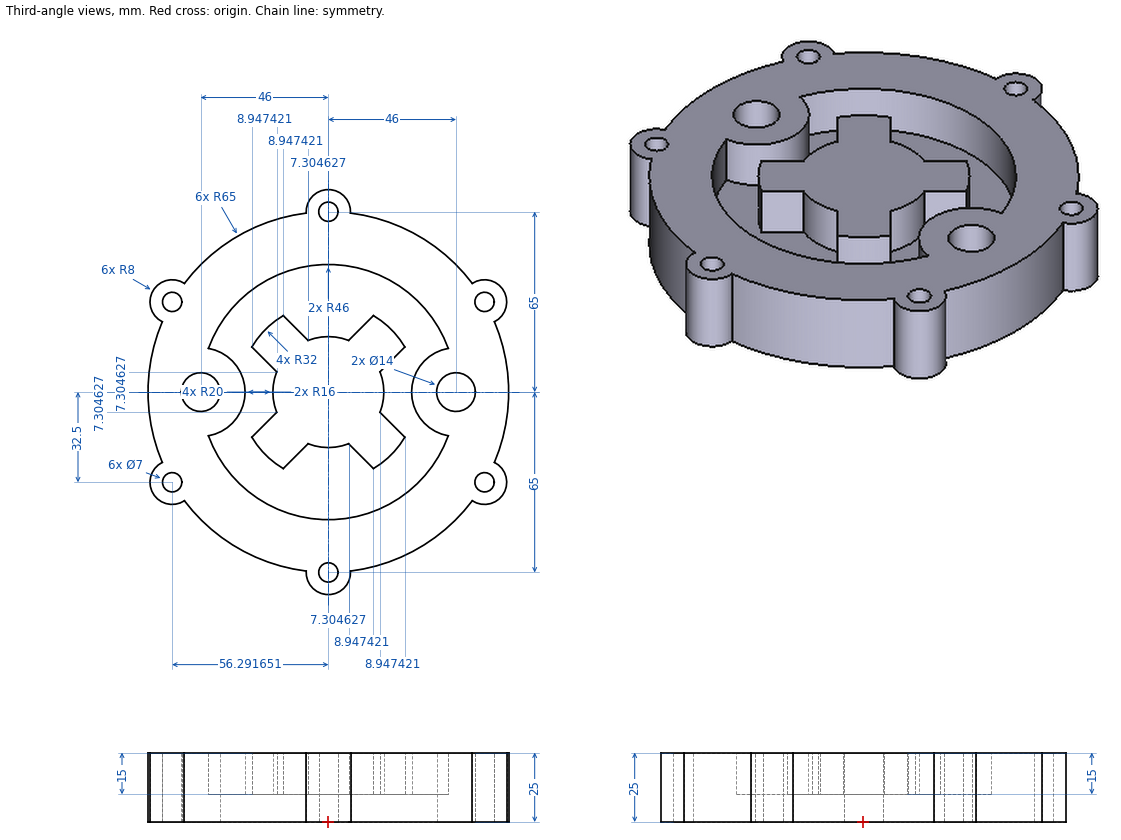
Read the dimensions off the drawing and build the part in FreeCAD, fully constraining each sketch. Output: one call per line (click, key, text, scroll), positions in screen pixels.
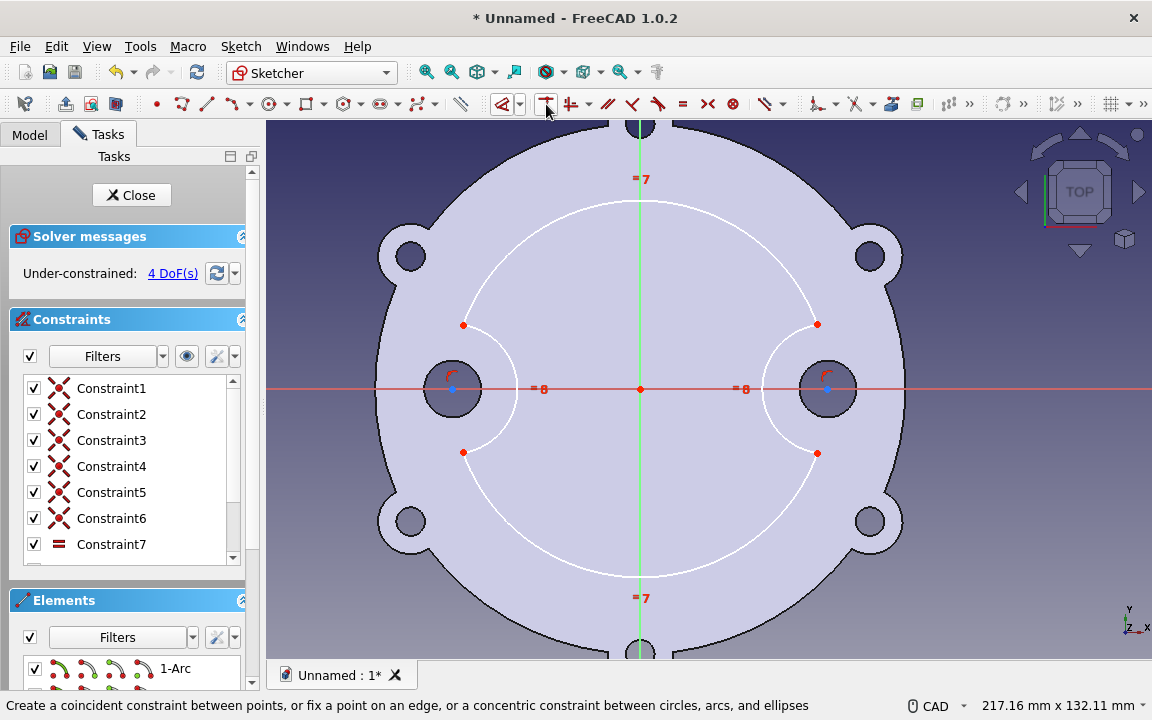
click(729, 223)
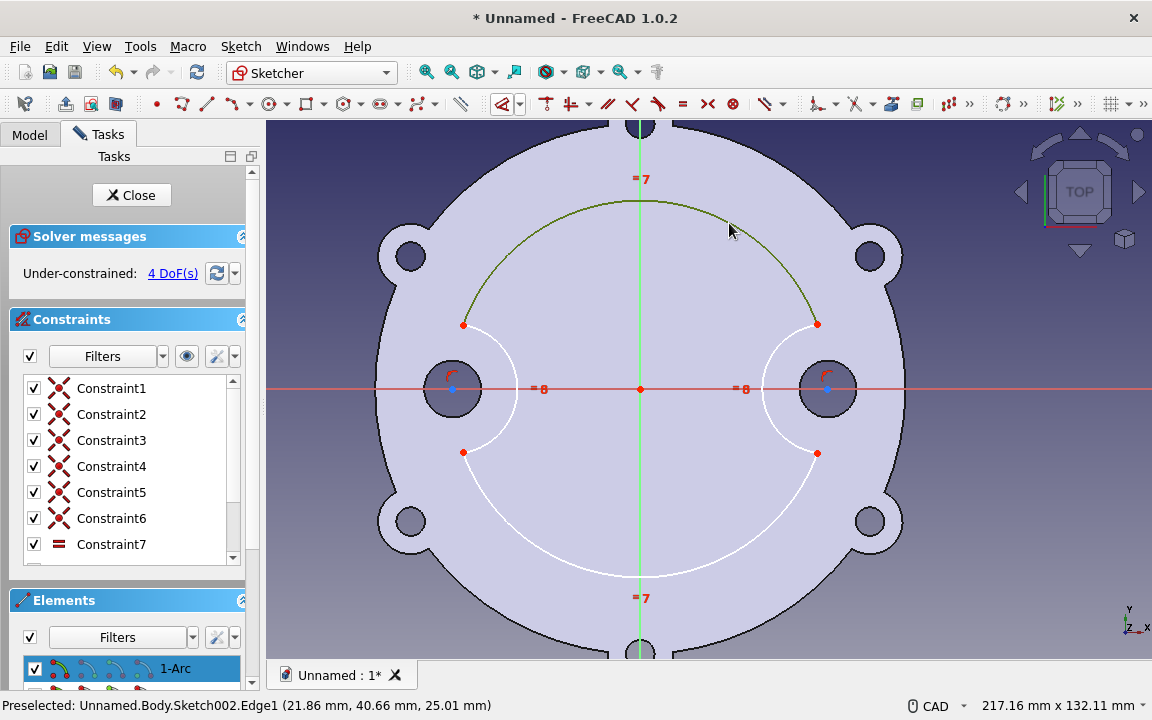
click(520, 104)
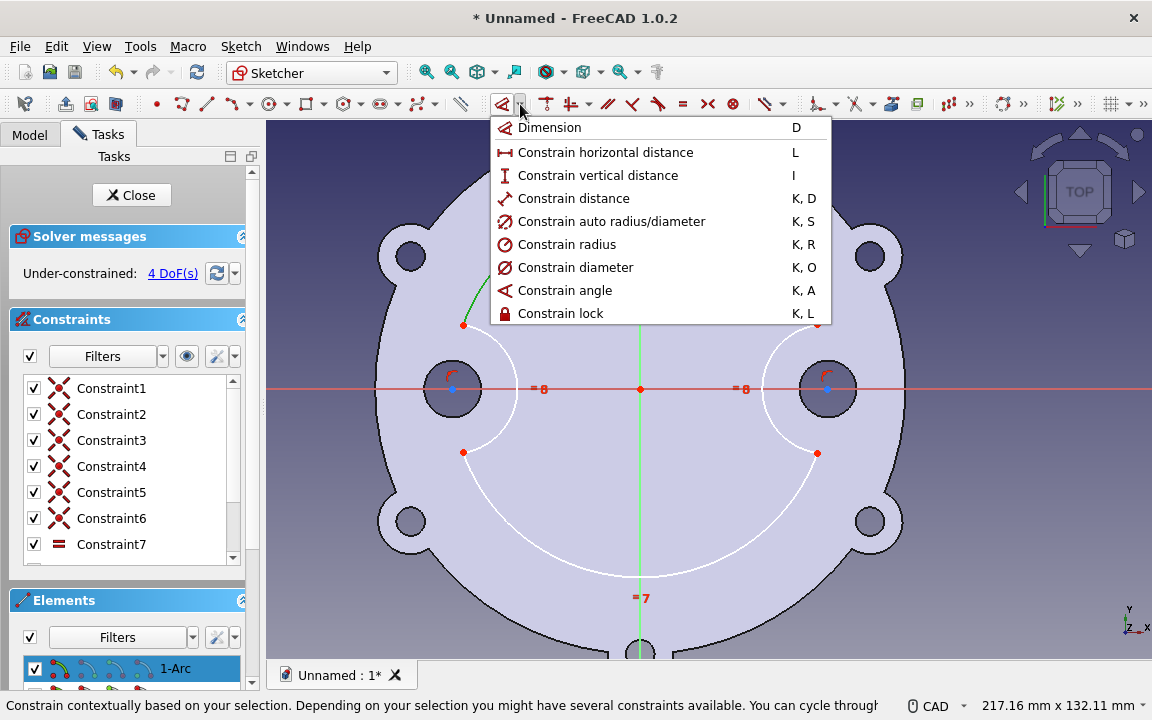
click(661, 244)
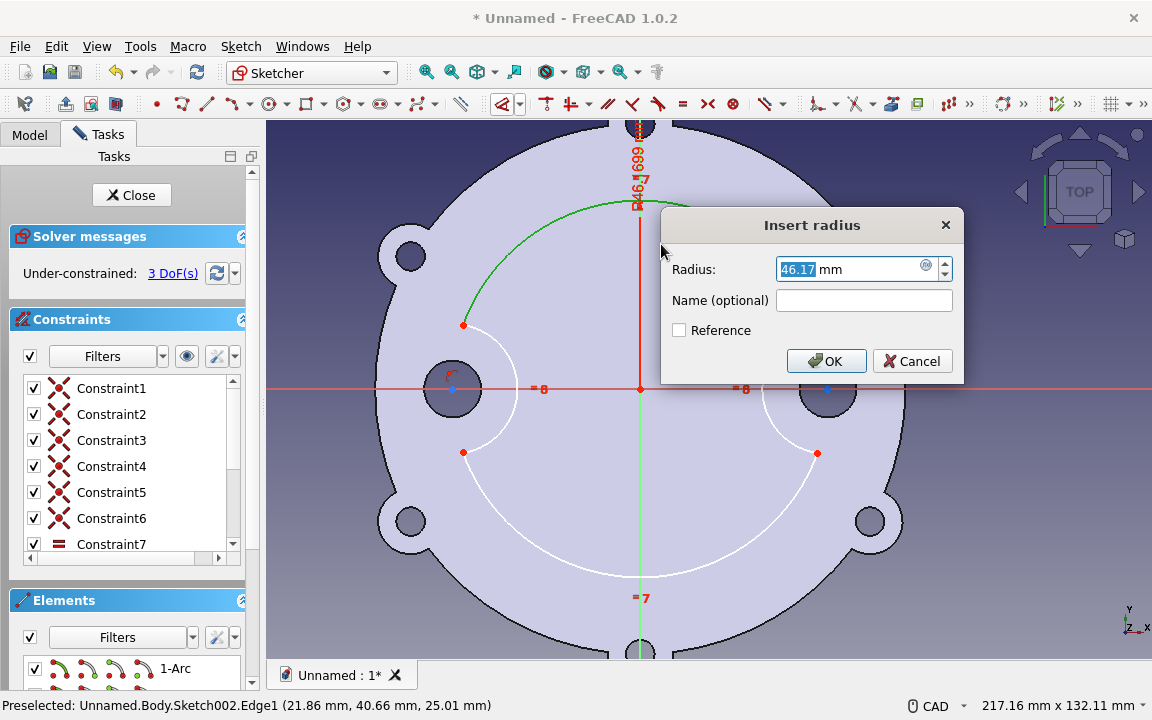
text(46)
key(Return)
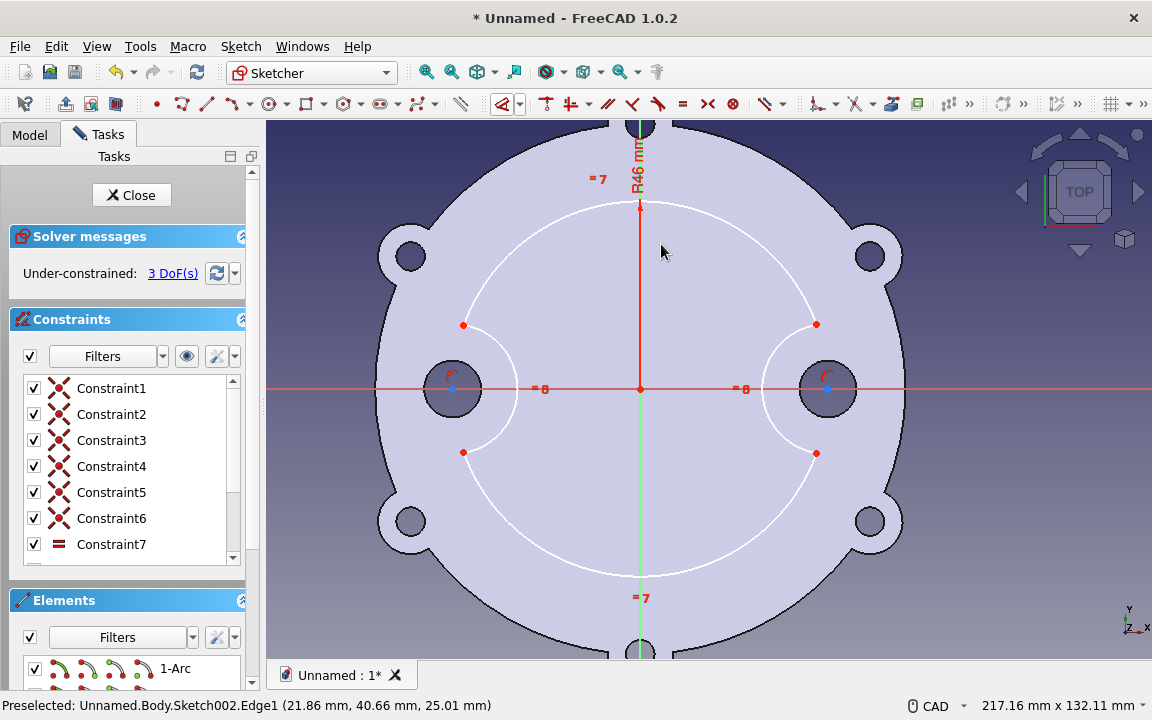
click(508, 423)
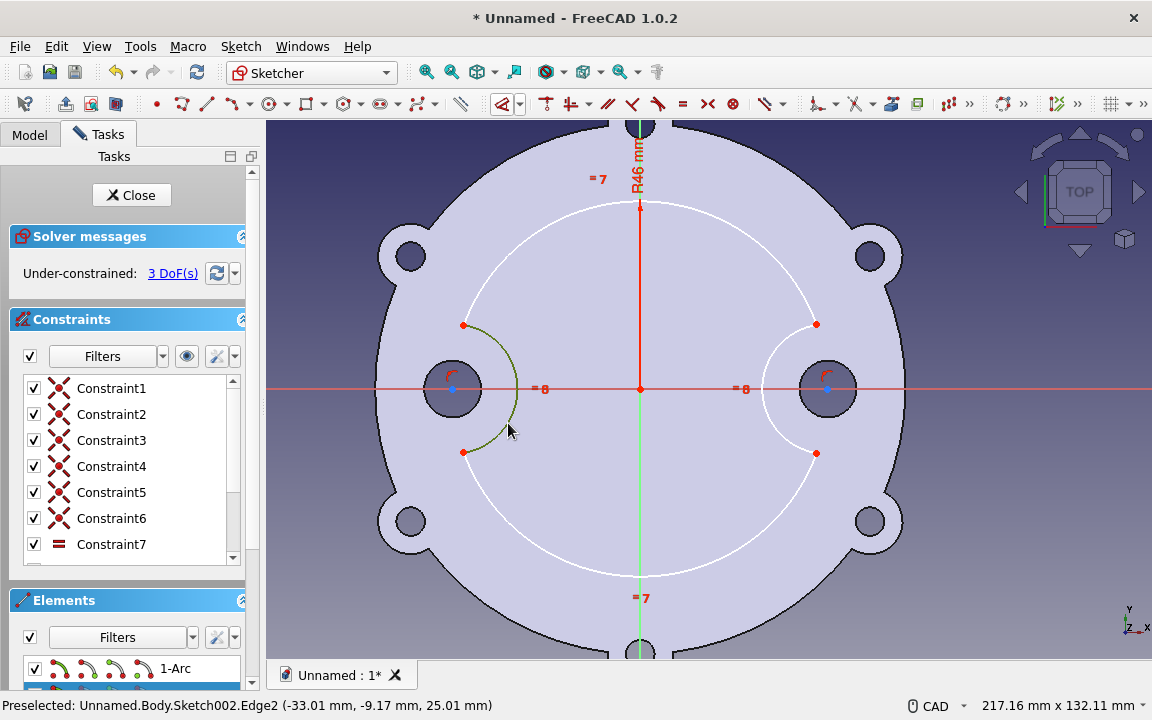
click(520, 104)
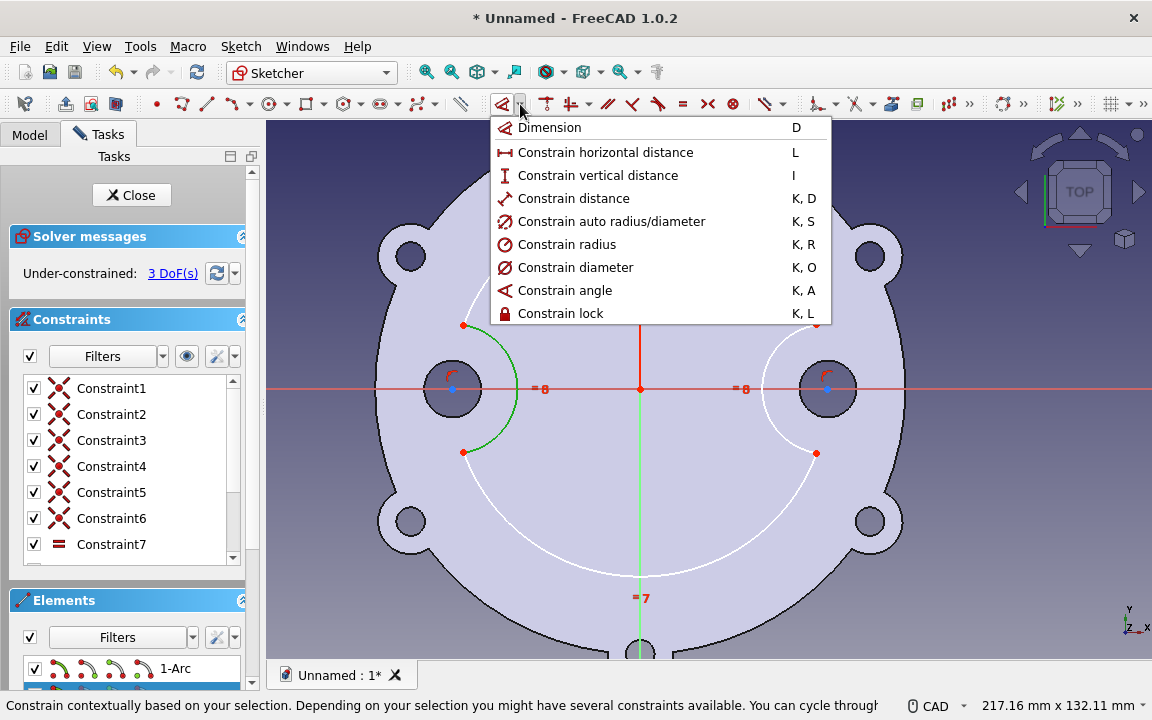
click(661, 244)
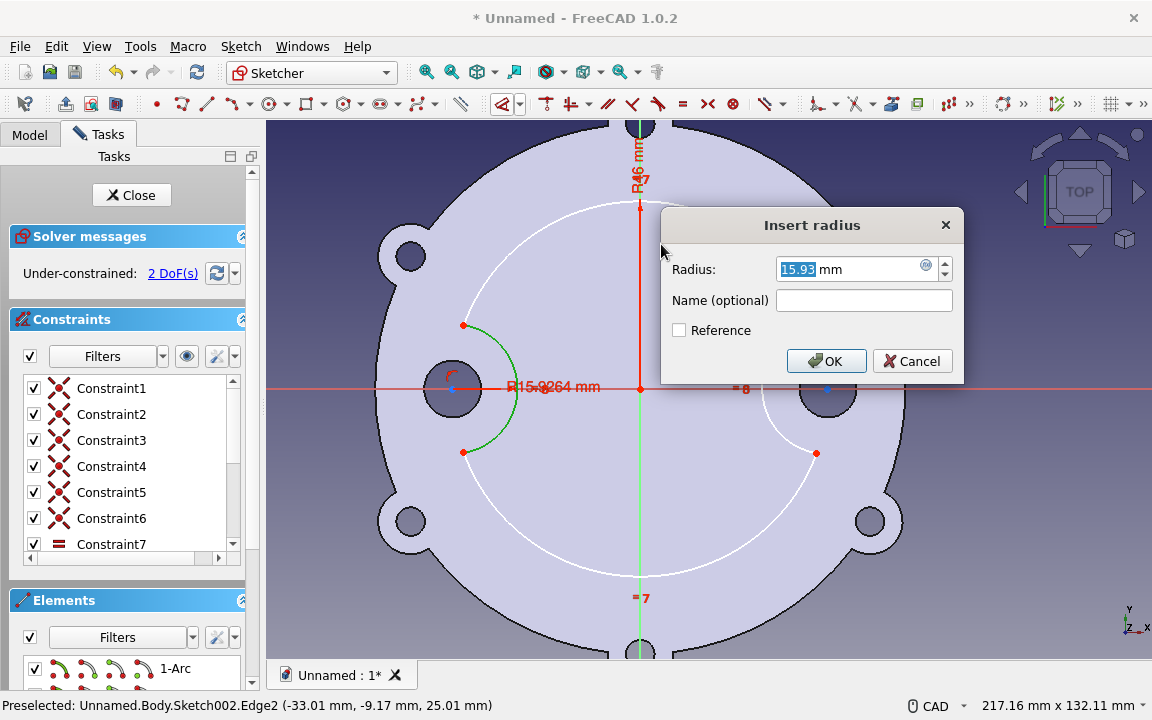
text(16)
key(Return)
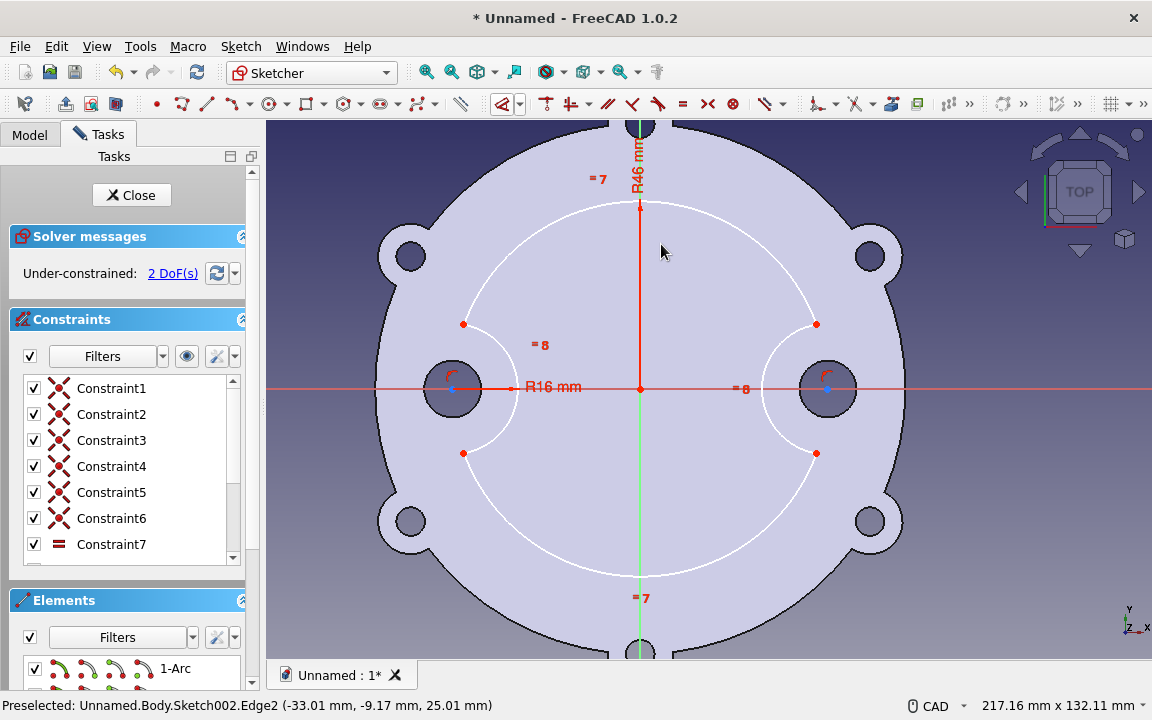
click(453, 389)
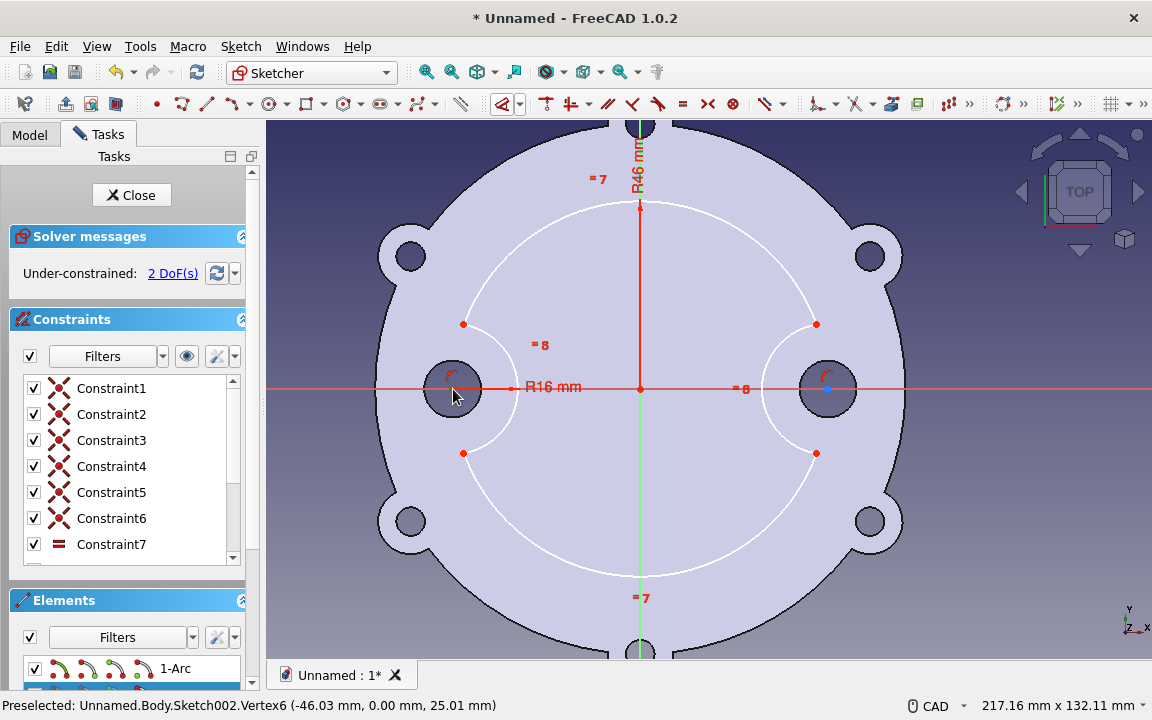
click(520, 104)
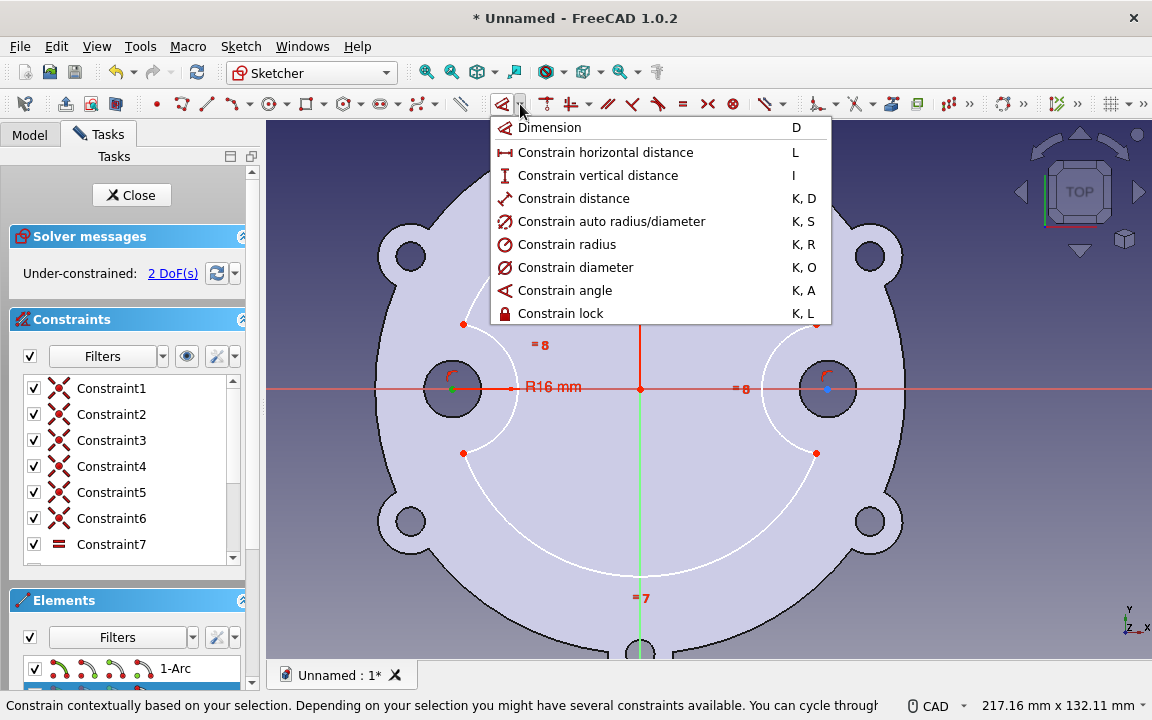
click(661, 152)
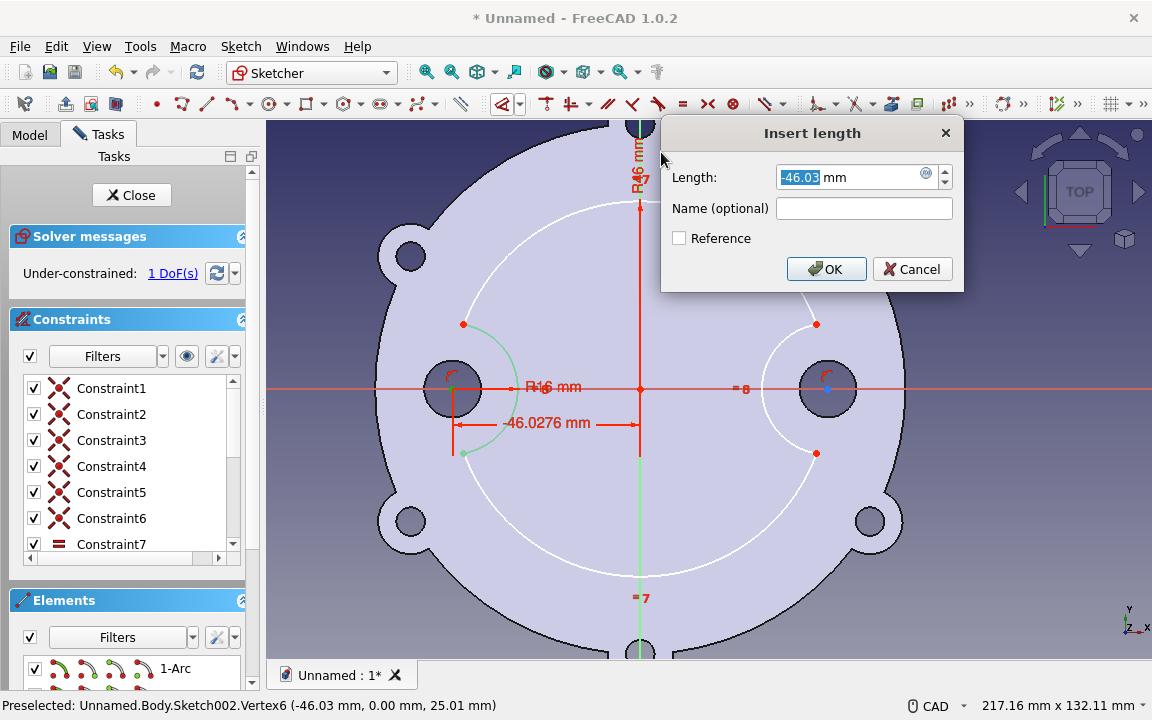
text(-46)
key(Return)